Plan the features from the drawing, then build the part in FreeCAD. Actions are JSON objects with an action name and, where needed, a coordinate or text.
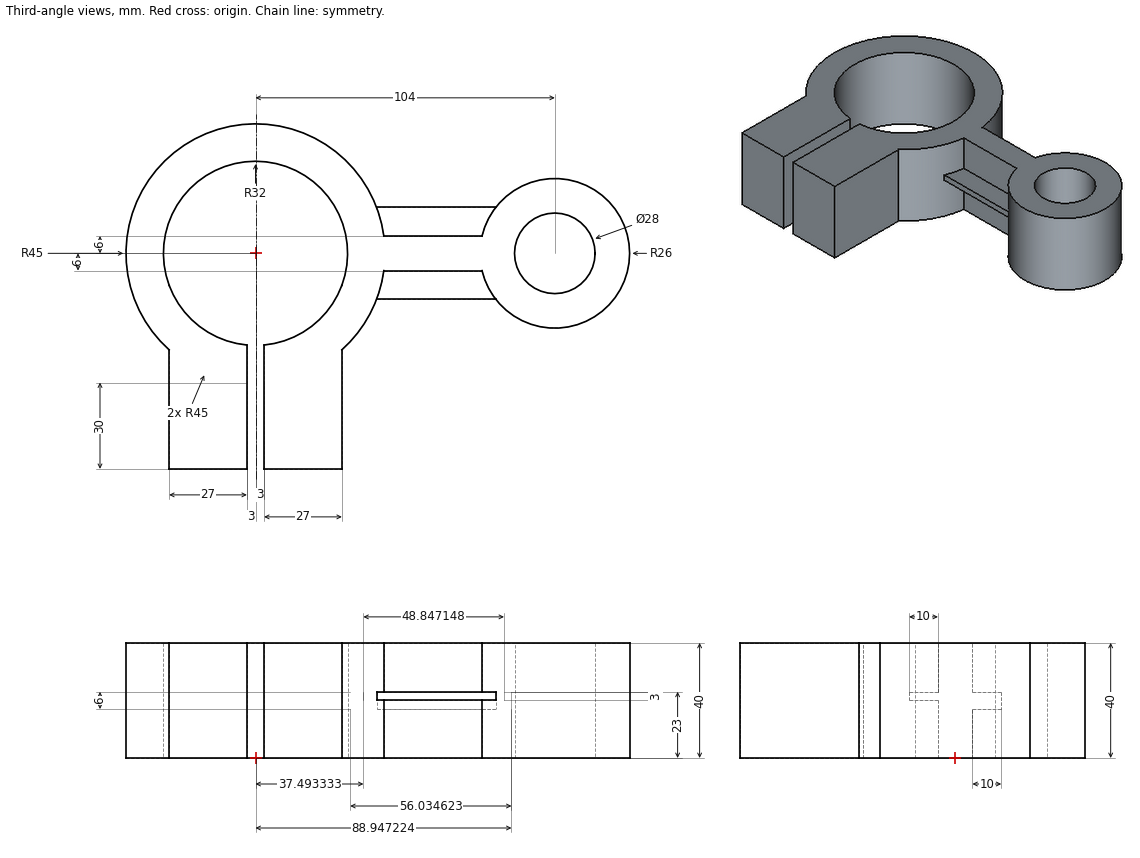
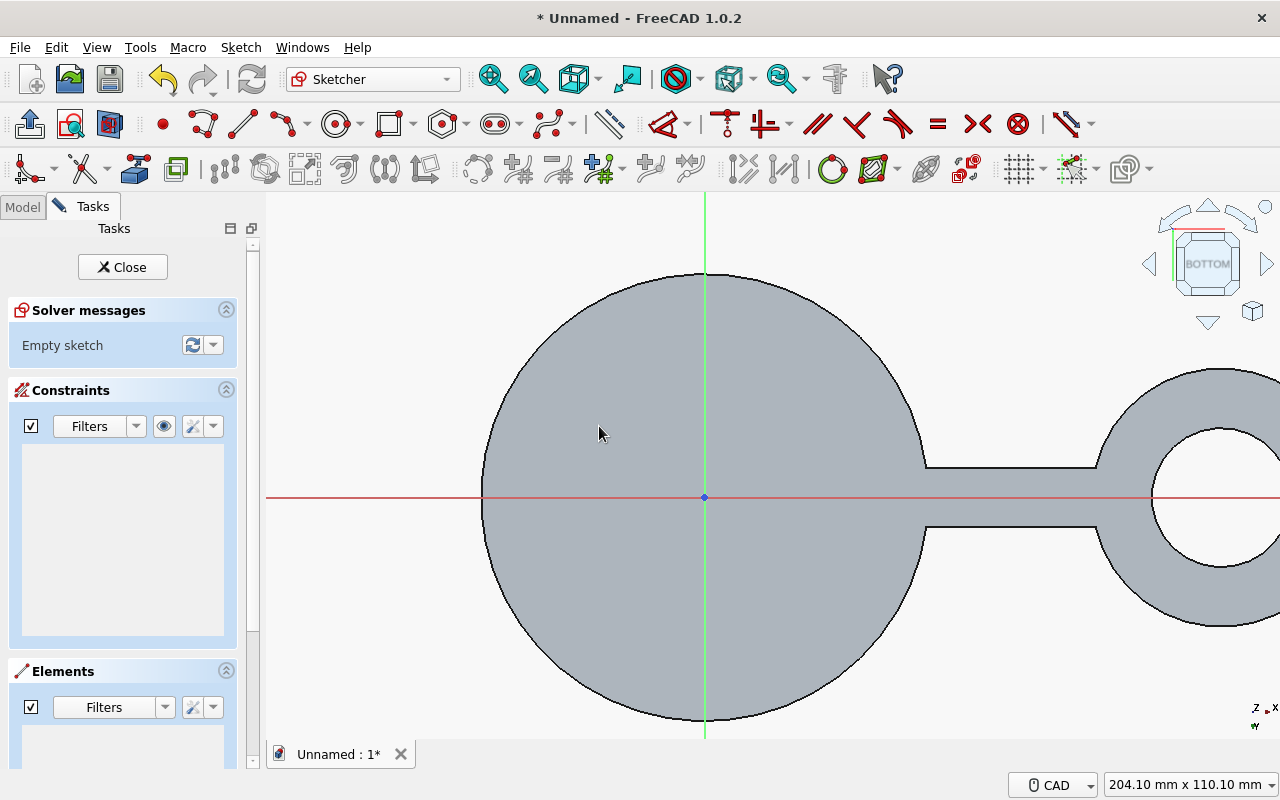
{"action": "key", "text": "g l"}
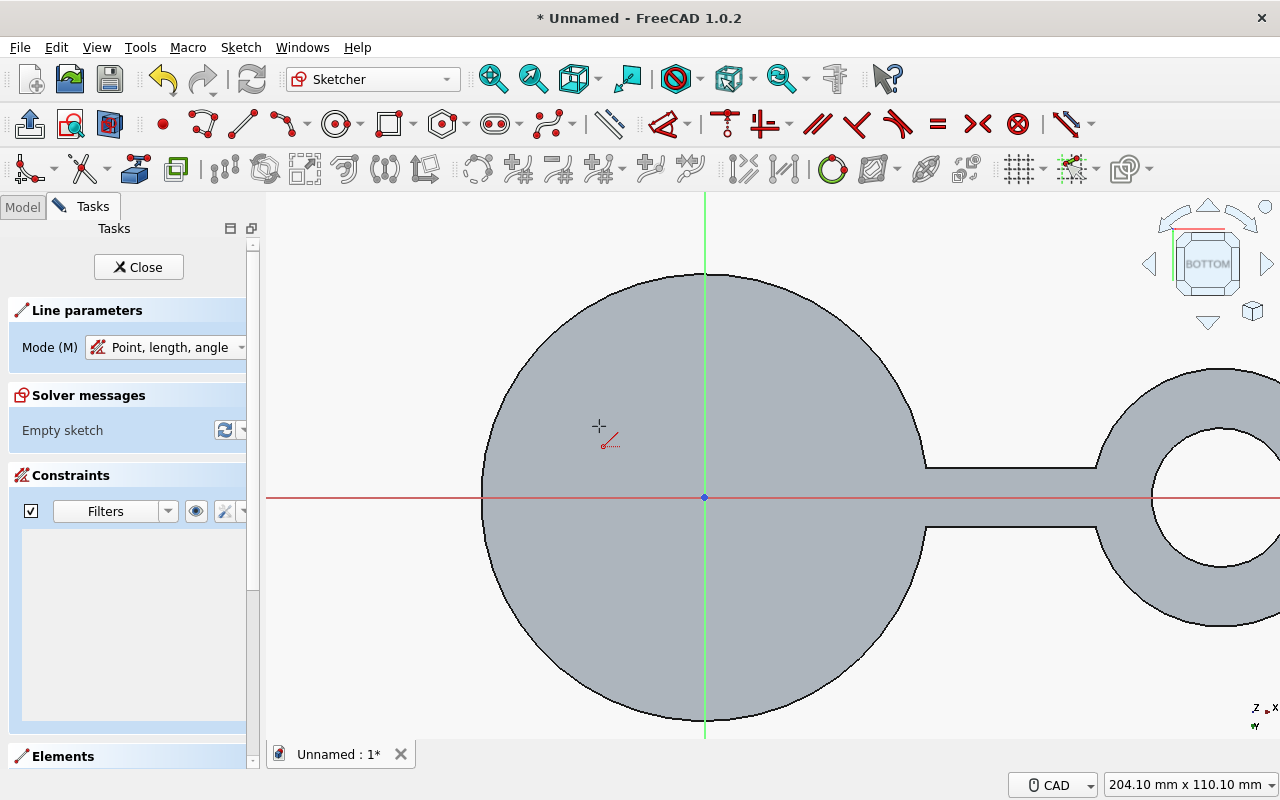
{"action": "left_click", "coordinate": [720, 275]}
{"action": "left_click", "coordinate": [720, 339]}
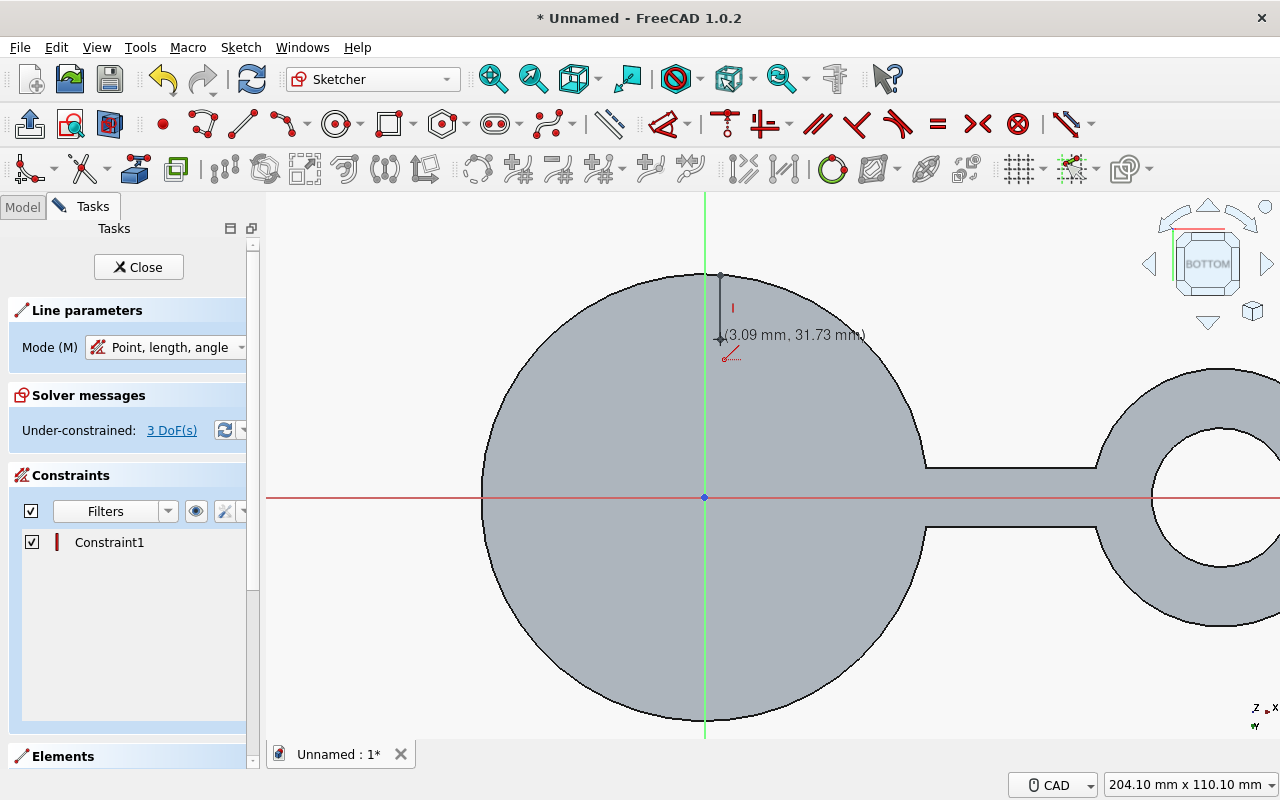
{"action": "left_click", "coordinate": [690, 339]}
{"action": "left_click", "coordinate": [690, 275]}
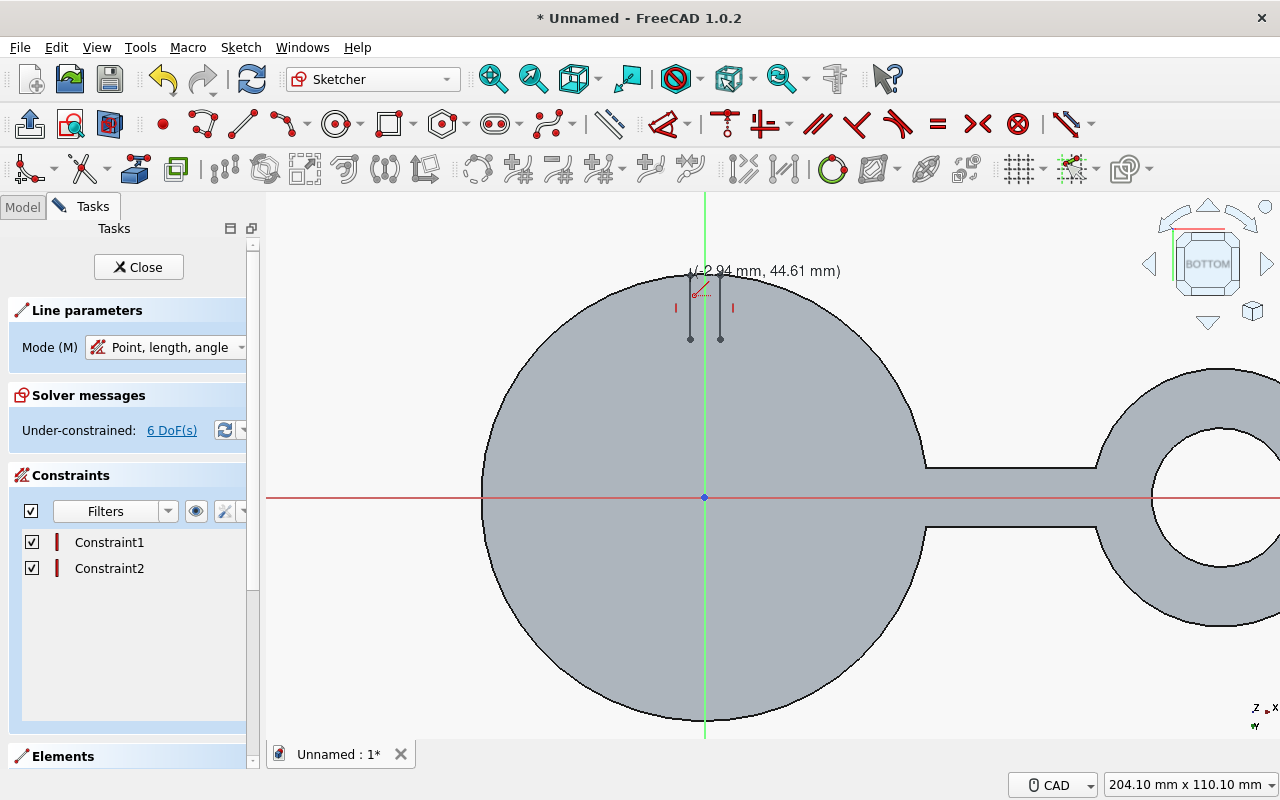
{"action": "key", "text": "g 3 a"}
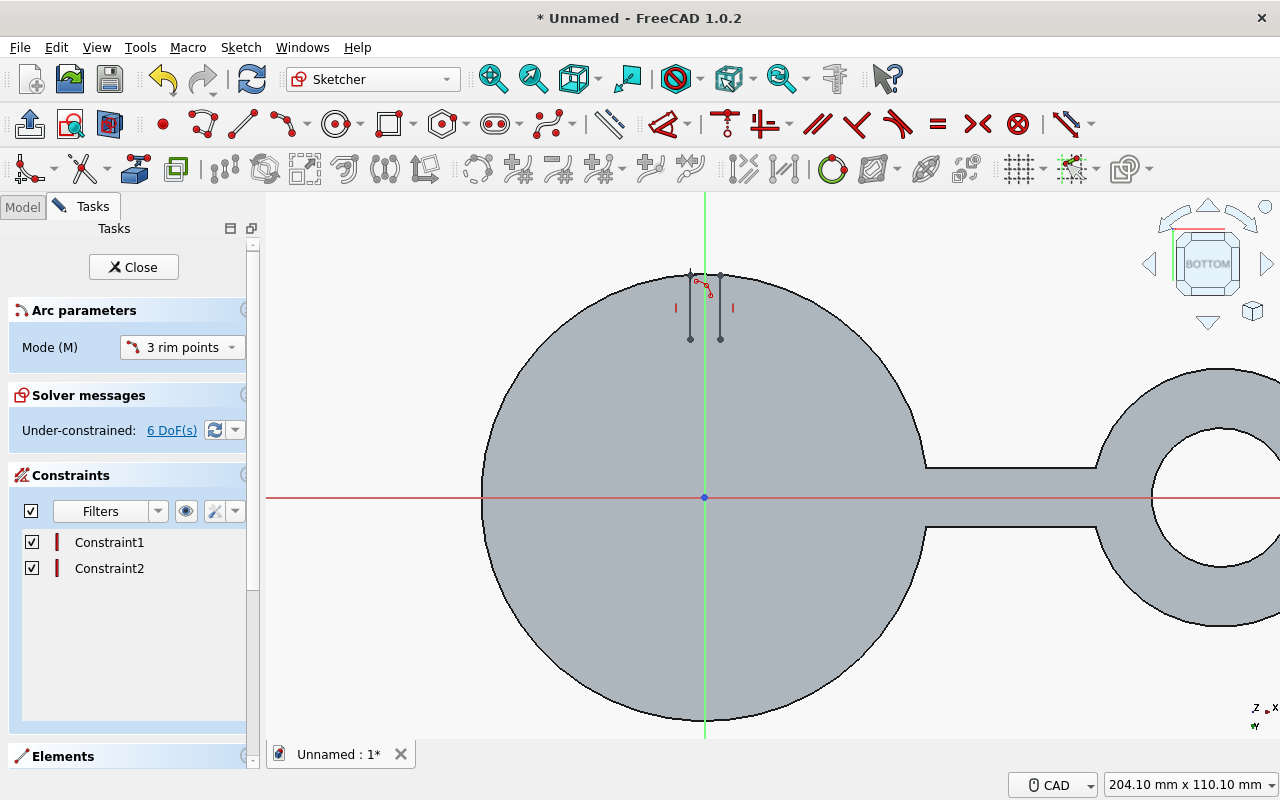
{"action": "left_click", "coordinate": [720, 340]}
{"action": "left_click", "coordinate": [690, 340]}
{"action": "left_click", "coordinate": [614, 628]}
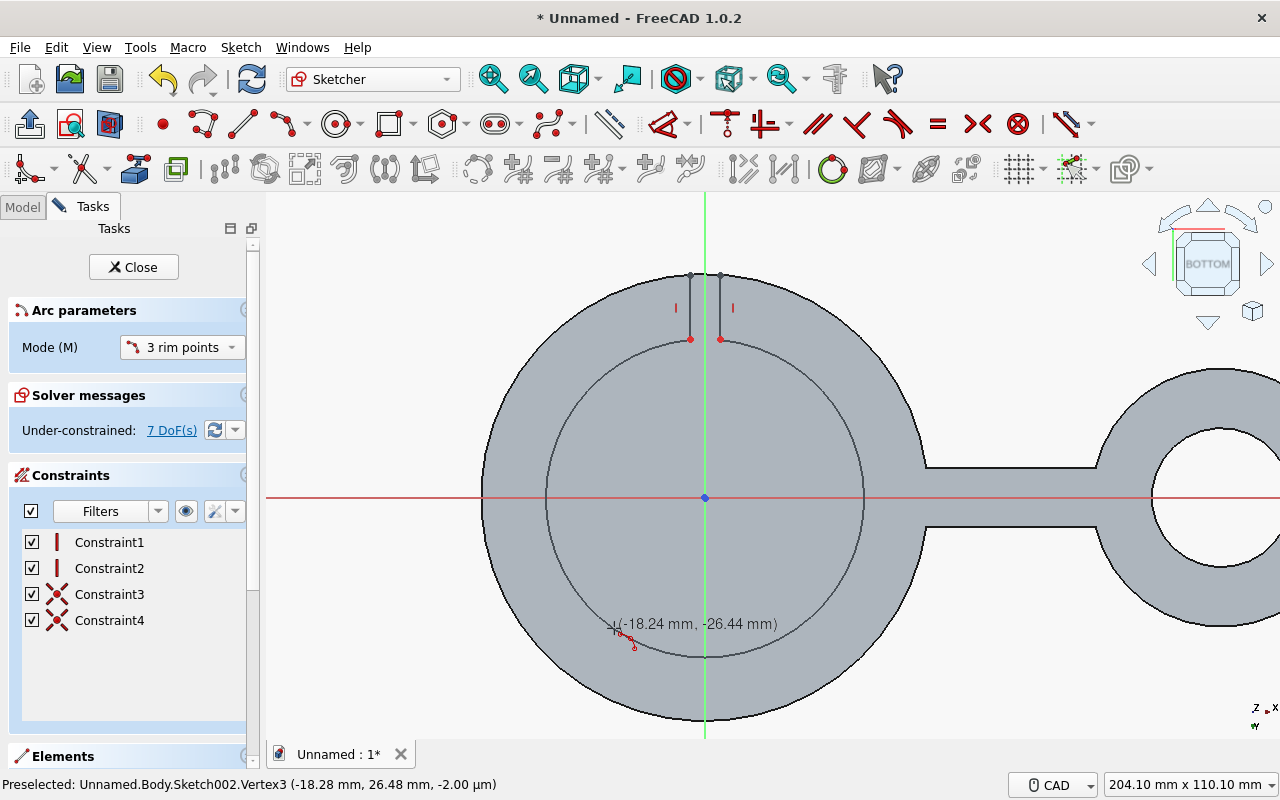
{"action": "left_click", "coordinate": [690, 276]}
{"action": "left_click", "coordinate": [720, 276]}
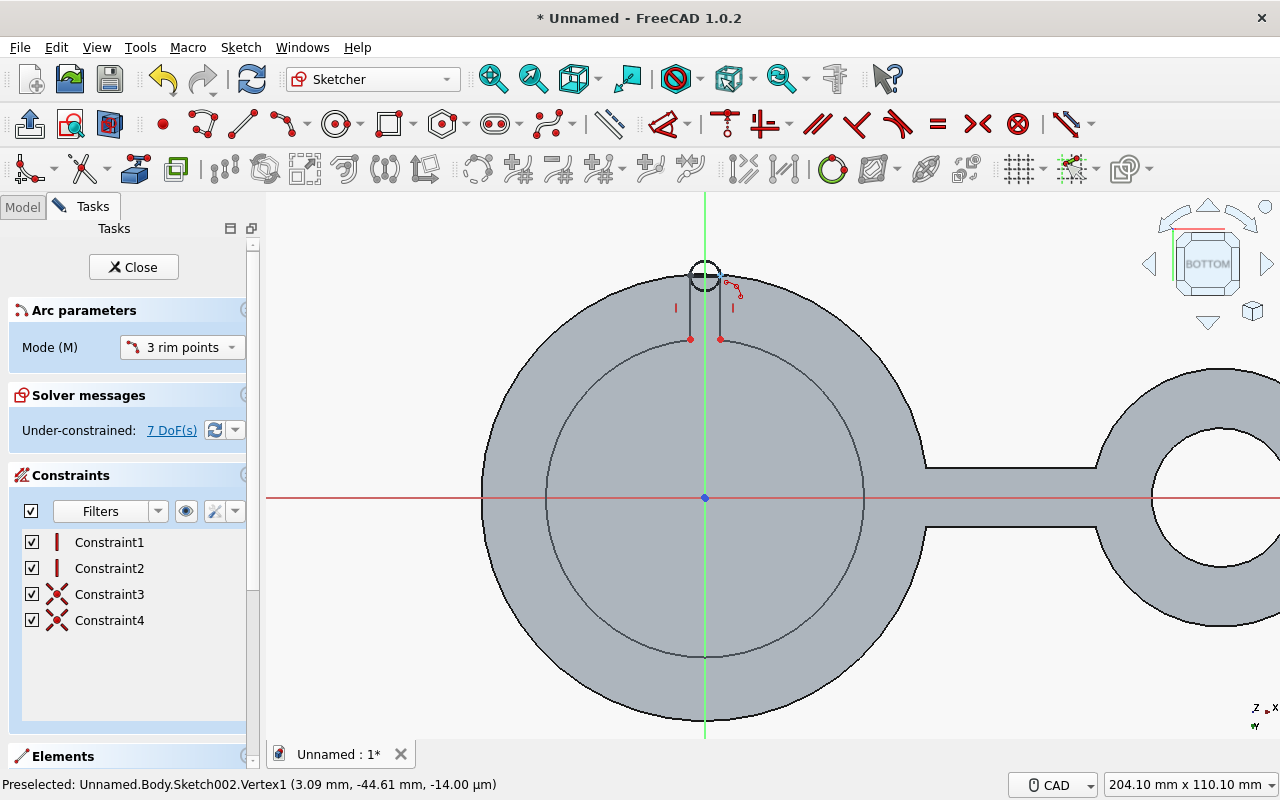
{"action": "scroll", "coordinate": [708, 274], "scroll_direction": "up", "scroll_amount": 18}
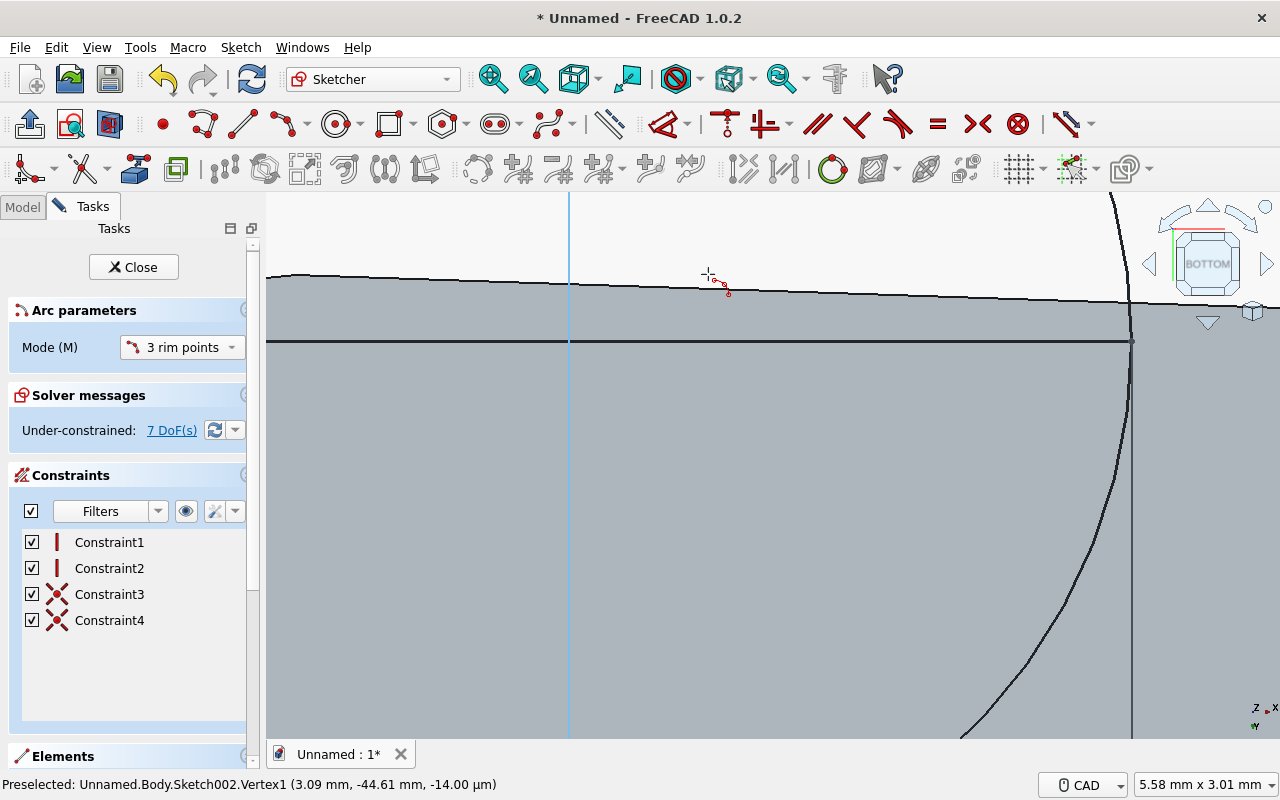
{"action": "left_click", "coordinate": [678, 271]}
{"action": "key", "text": "Escape"}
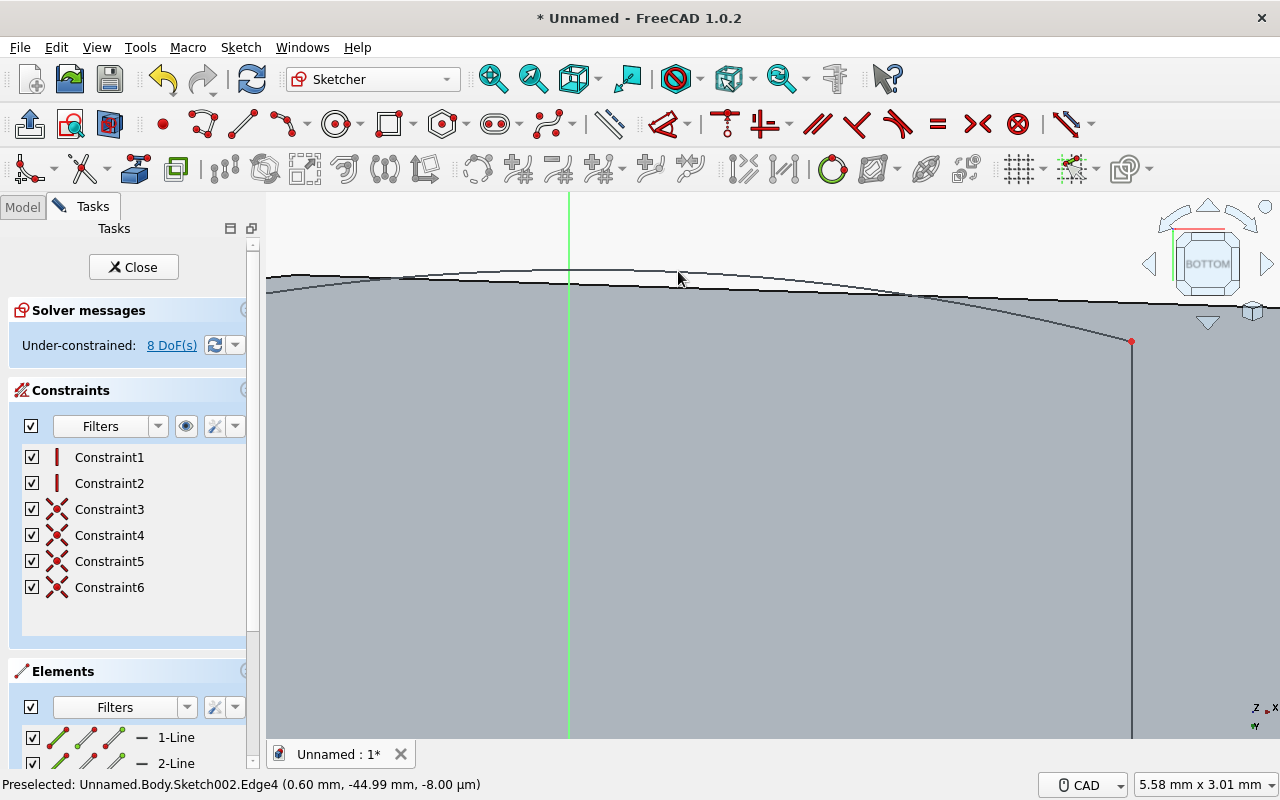
{"action": "scroll", "coordinate": [708, 274], "scroll_direction": "down", "scroll_amount": 18}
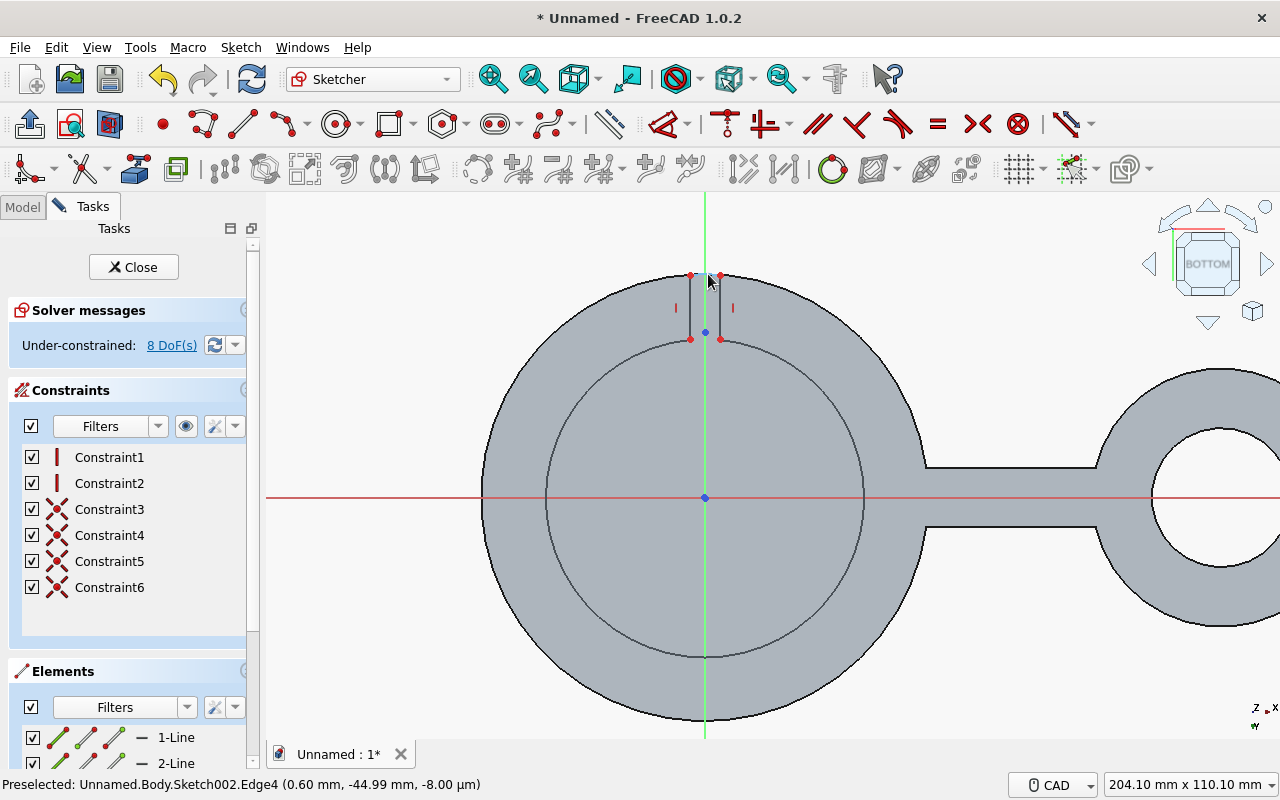
{"action": "left_click", "coordinate": [556, 553]}